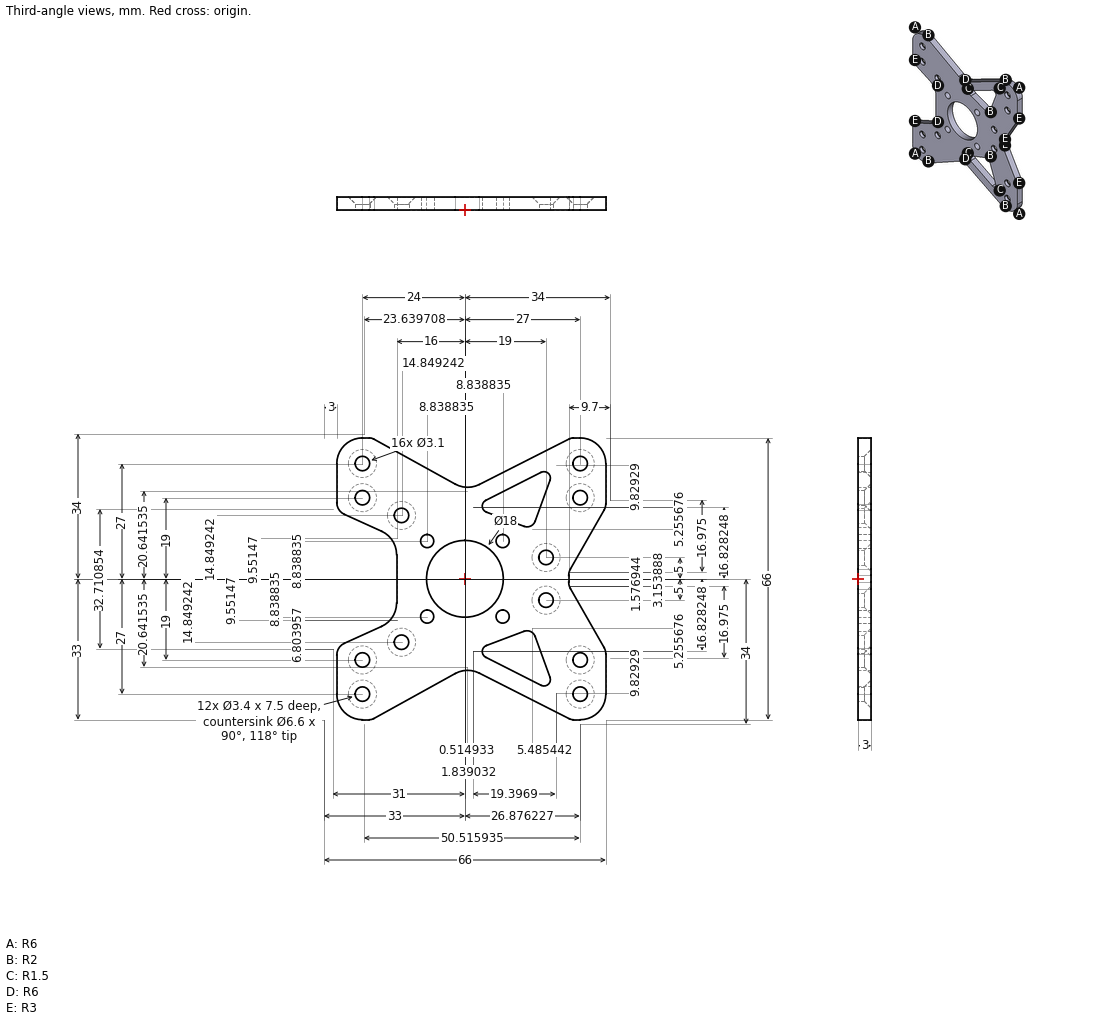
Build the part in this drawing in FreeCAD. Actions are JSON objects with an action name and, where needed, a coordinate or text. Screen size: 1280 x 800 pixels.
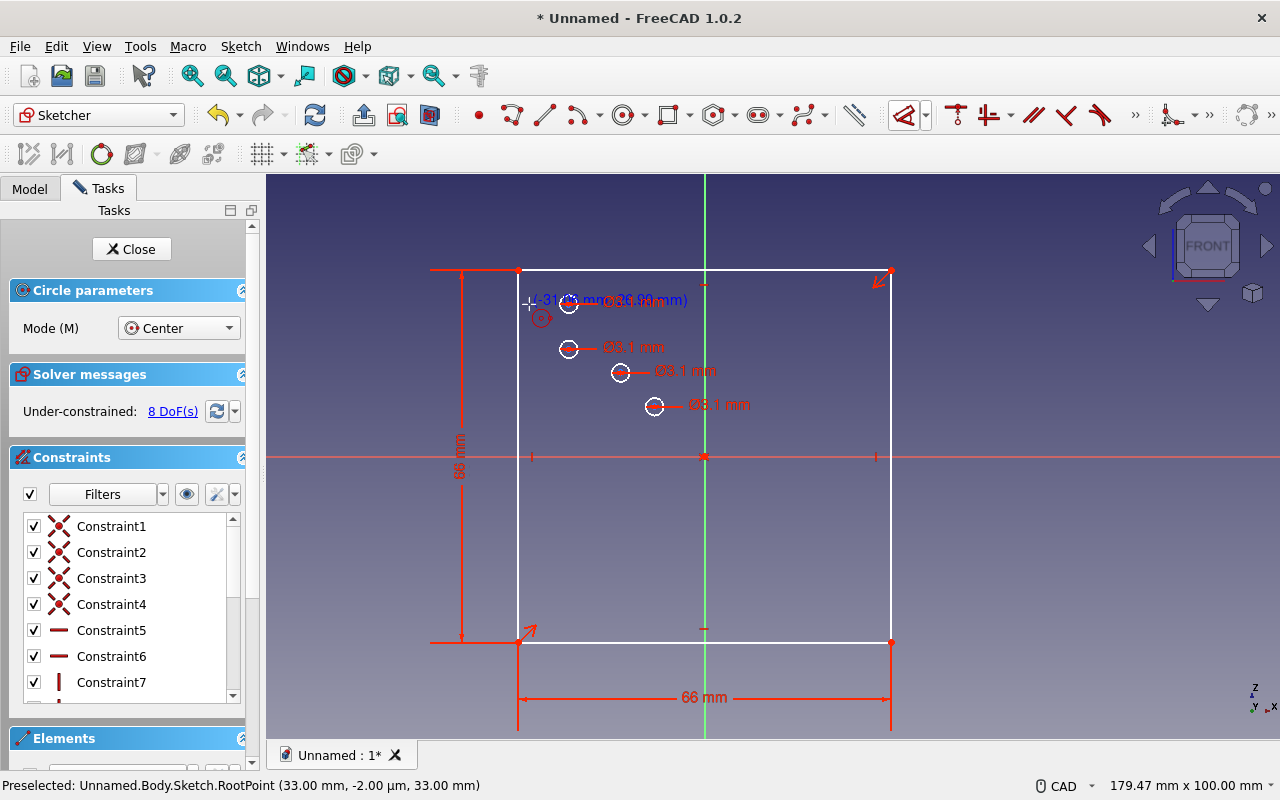
{"action": "scroll", "coordinate": [857, 304], "scroll_direction": "up", "scroll_amount": 5}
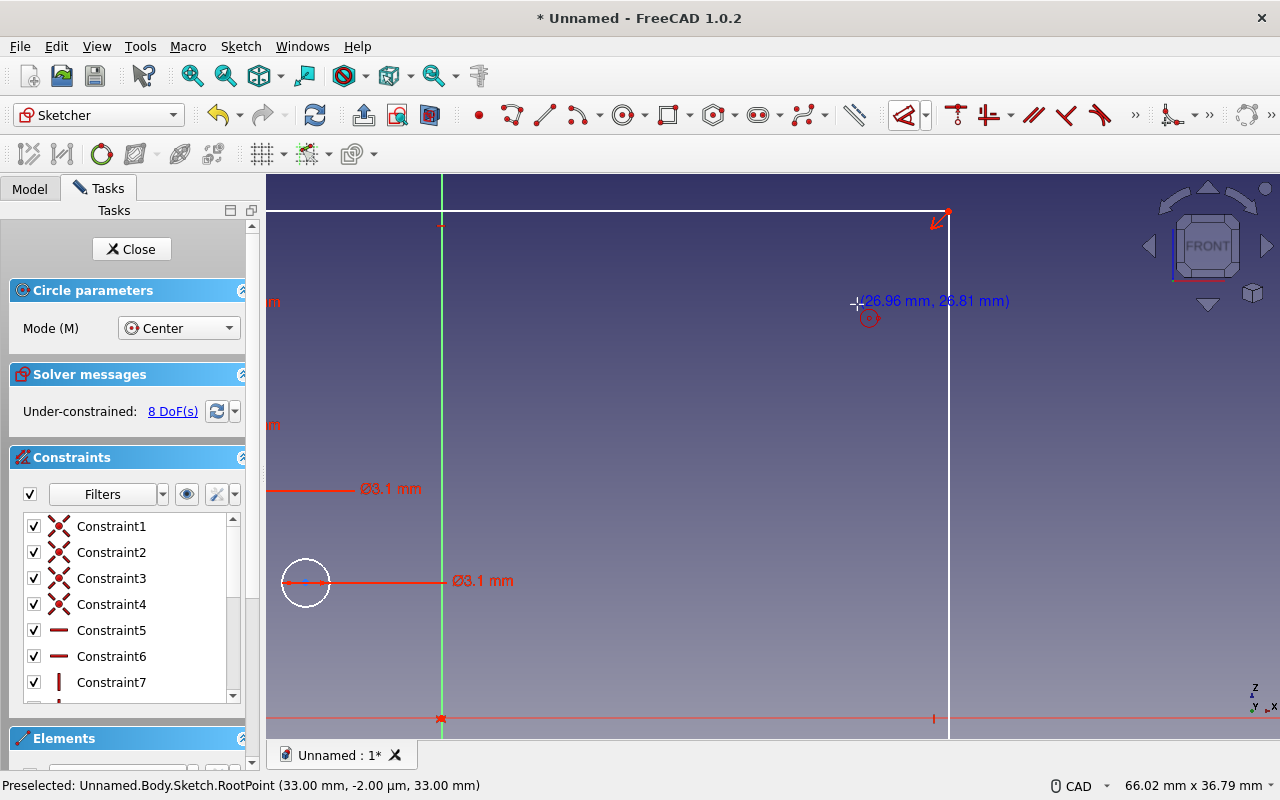
{"action": "left_click", "coordinate": [857, 303]}
{"action": "mouse_move", "coordinate": [873, 287]}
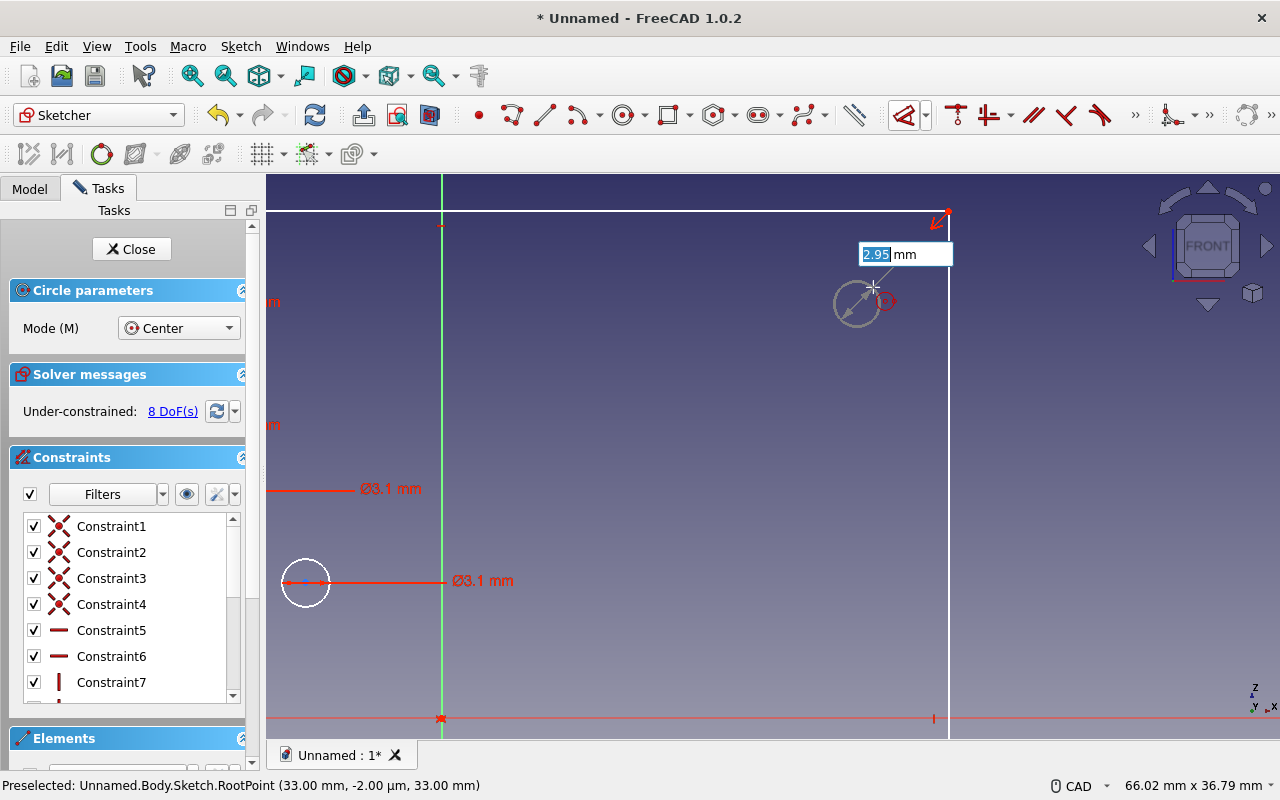
{"action": "type", "text": "3.1"}
{"action": "key", "text": "Return"}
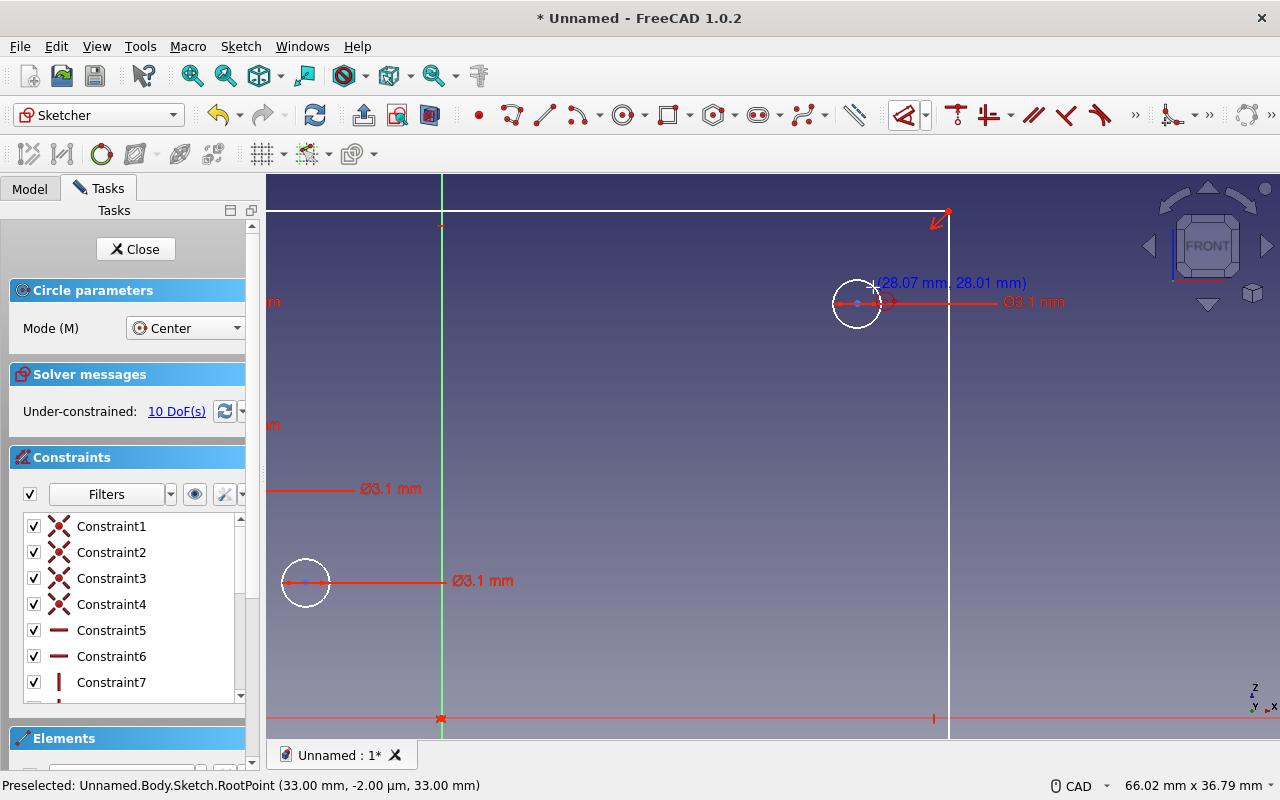
{"action": "left_click", "coordinate": [857, 426]}
{"action": "mouse_move", "coordinate": [873, 410]}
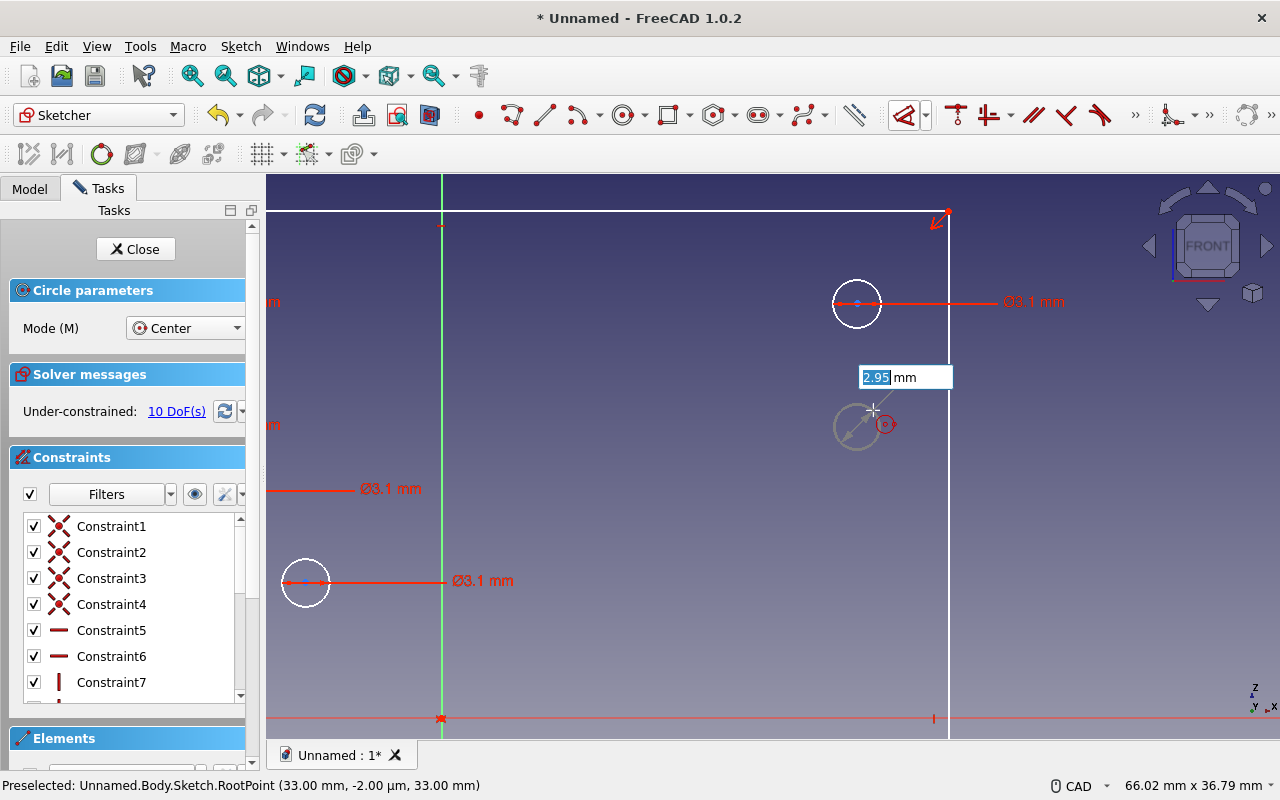
{"action": "type", "text": "3.1"}
{"action": "key", "text": "Return"}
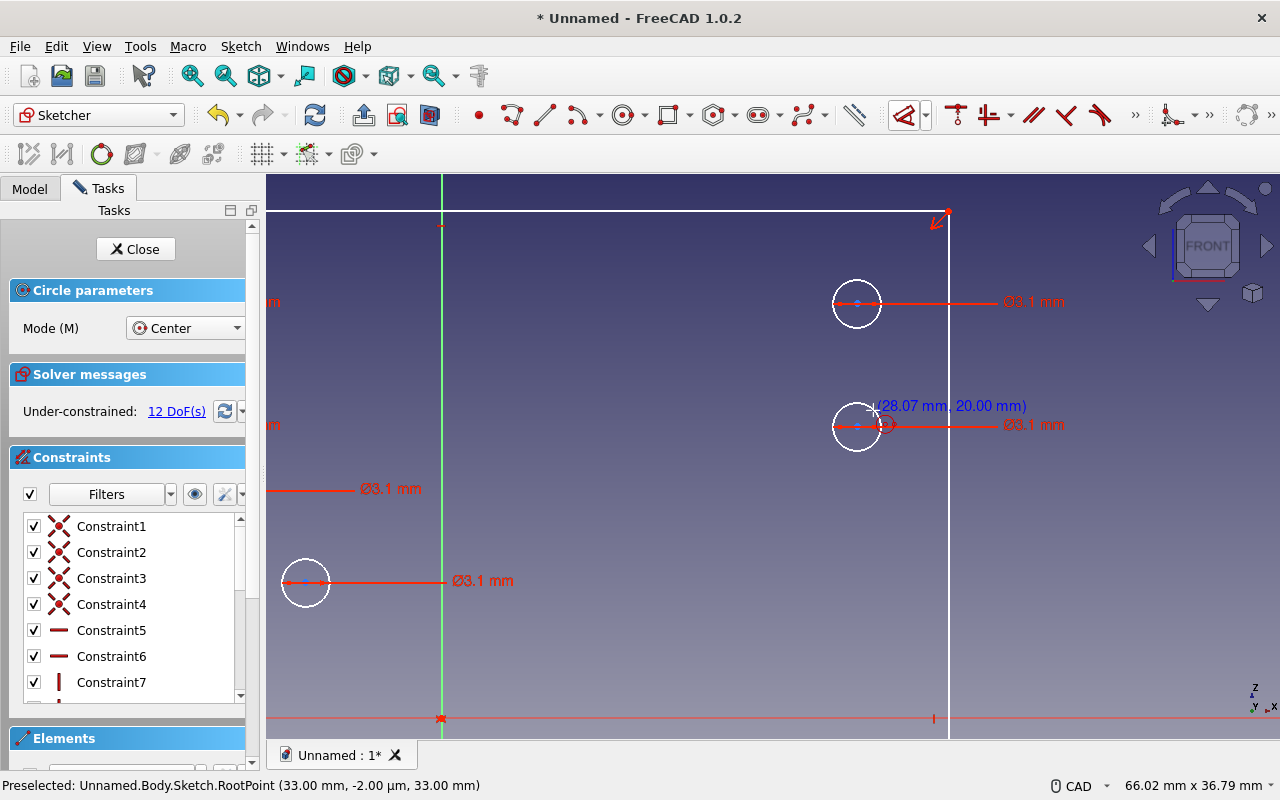
{"action": "left_click", "coordinate": [578, 582]}
{"action": "mouse_move", "coordinate": [594, 566]}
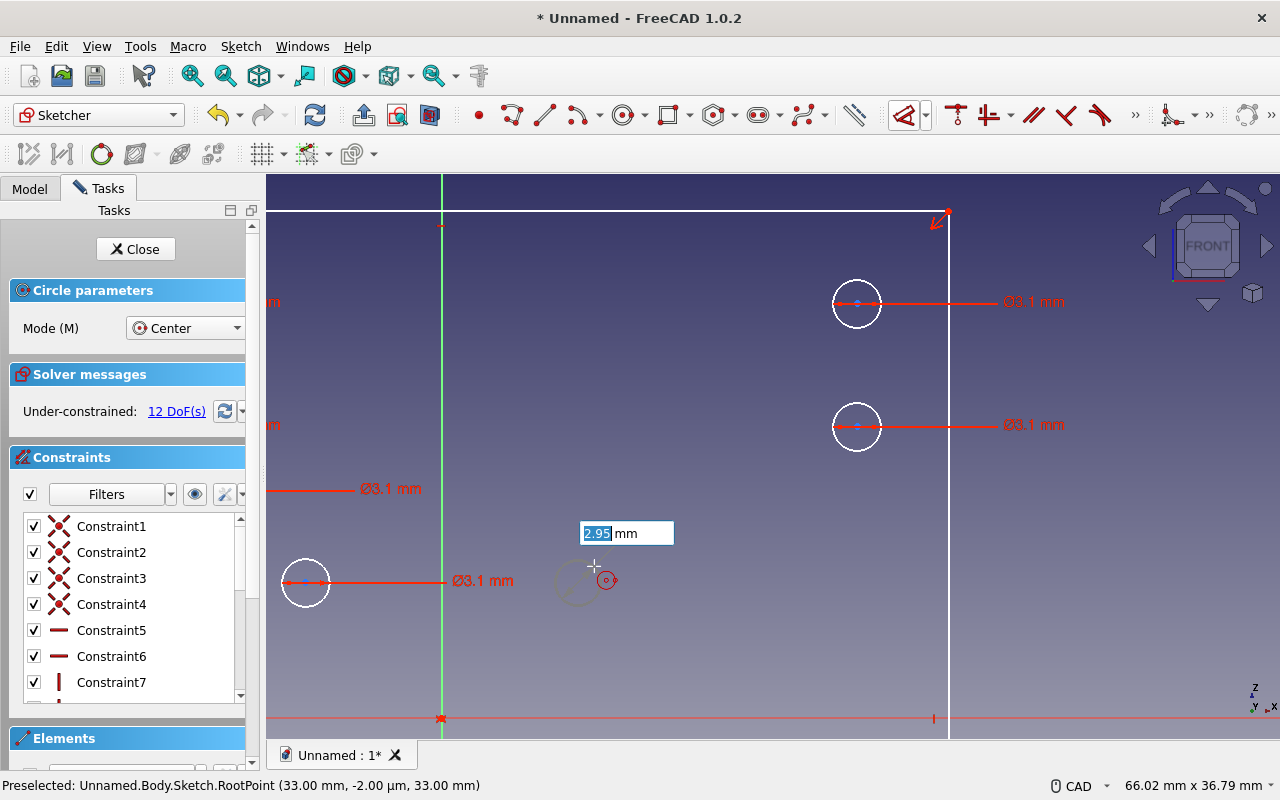
{"action": "type", "text": "3.1"}
{"action": "key", "text": "Return"}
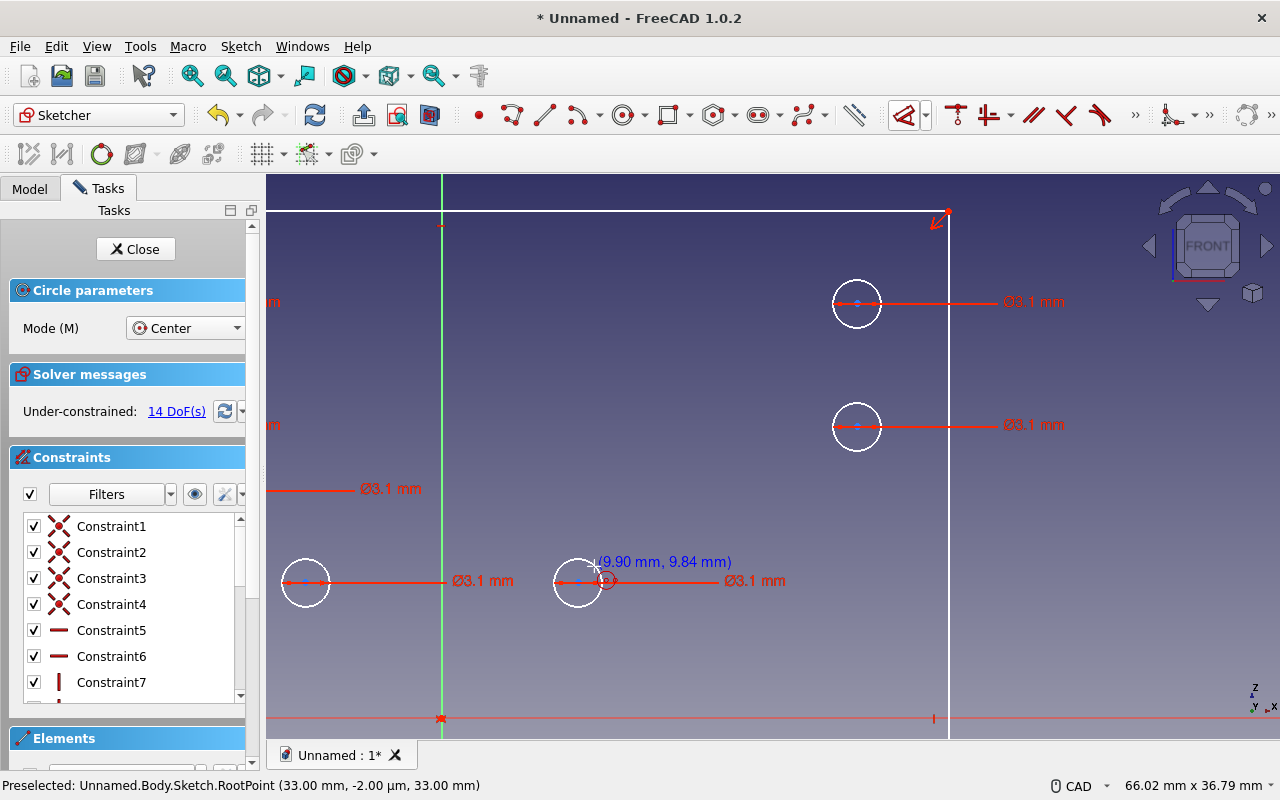
{"action": "left_click", "coordinate": [734, 641]}
{"action": "mouse_move", "coordinate": [751, 625]}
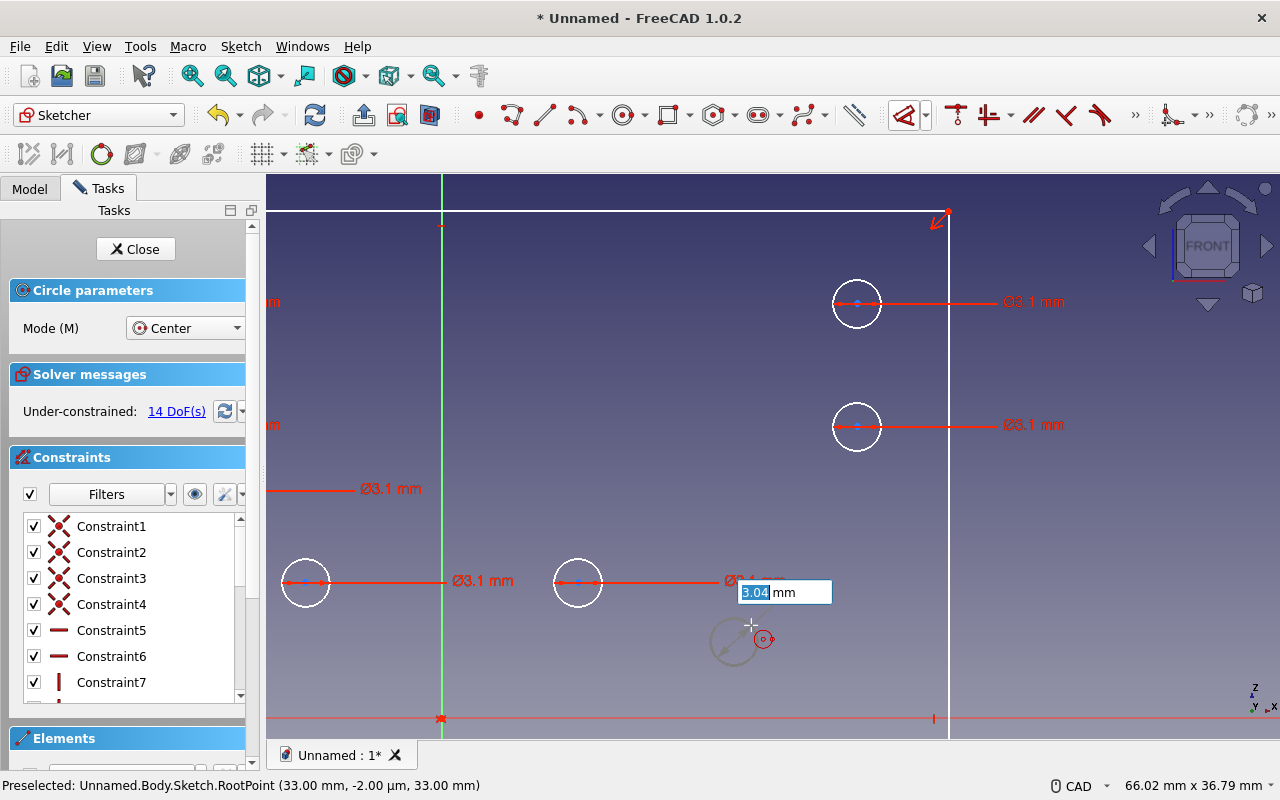
{"action": "type", "text": "3.1"}
{"action": "key", "text": "Return"}